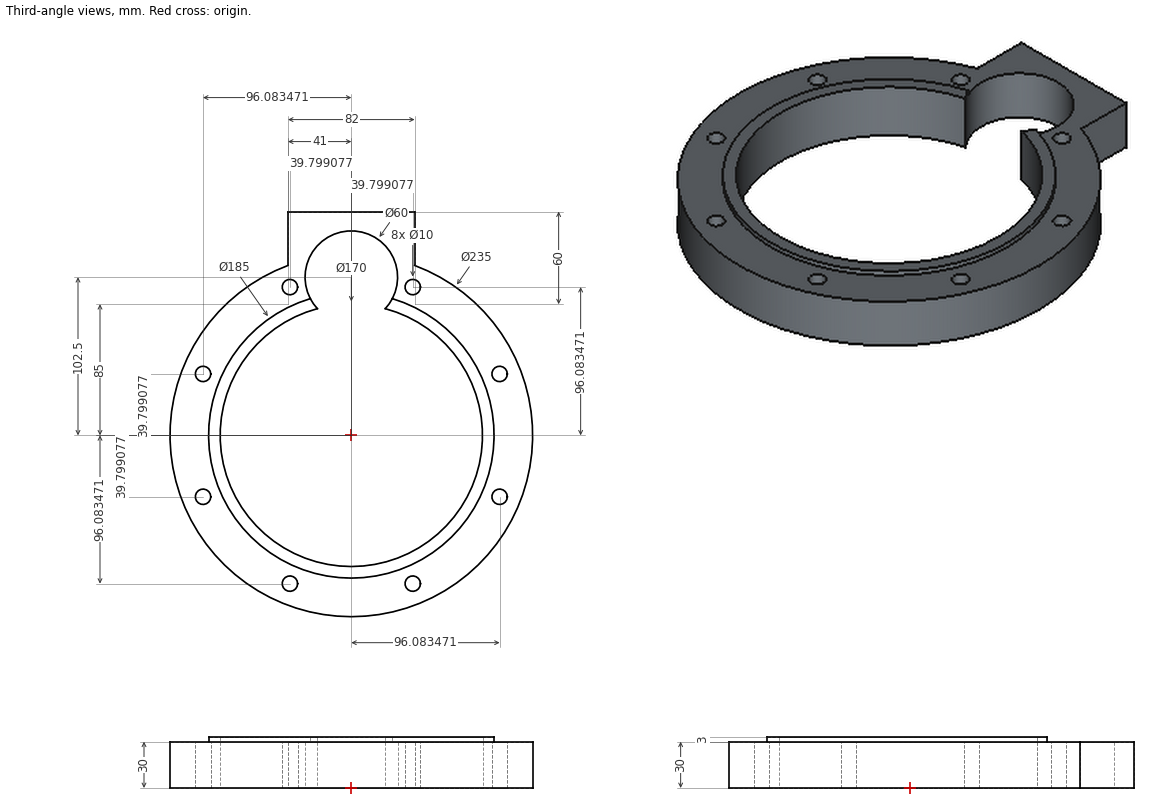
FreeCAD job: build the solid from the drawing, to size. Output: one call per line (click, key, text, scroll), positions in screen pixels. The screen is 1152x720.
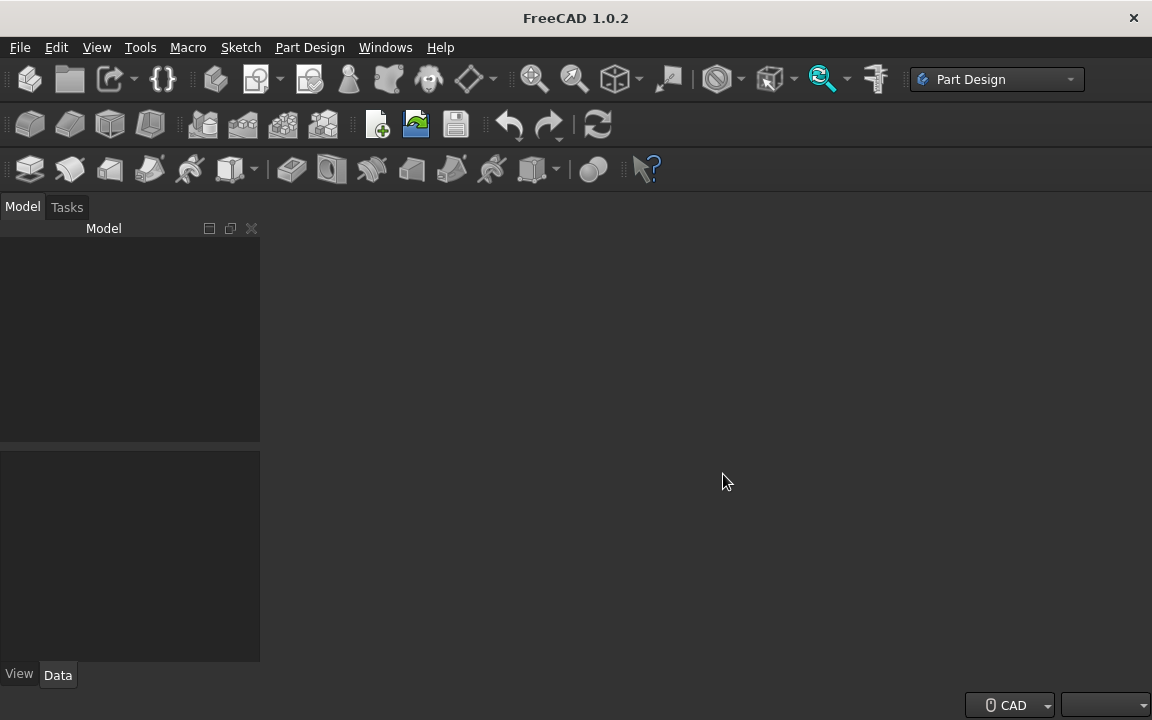
click(376, 124)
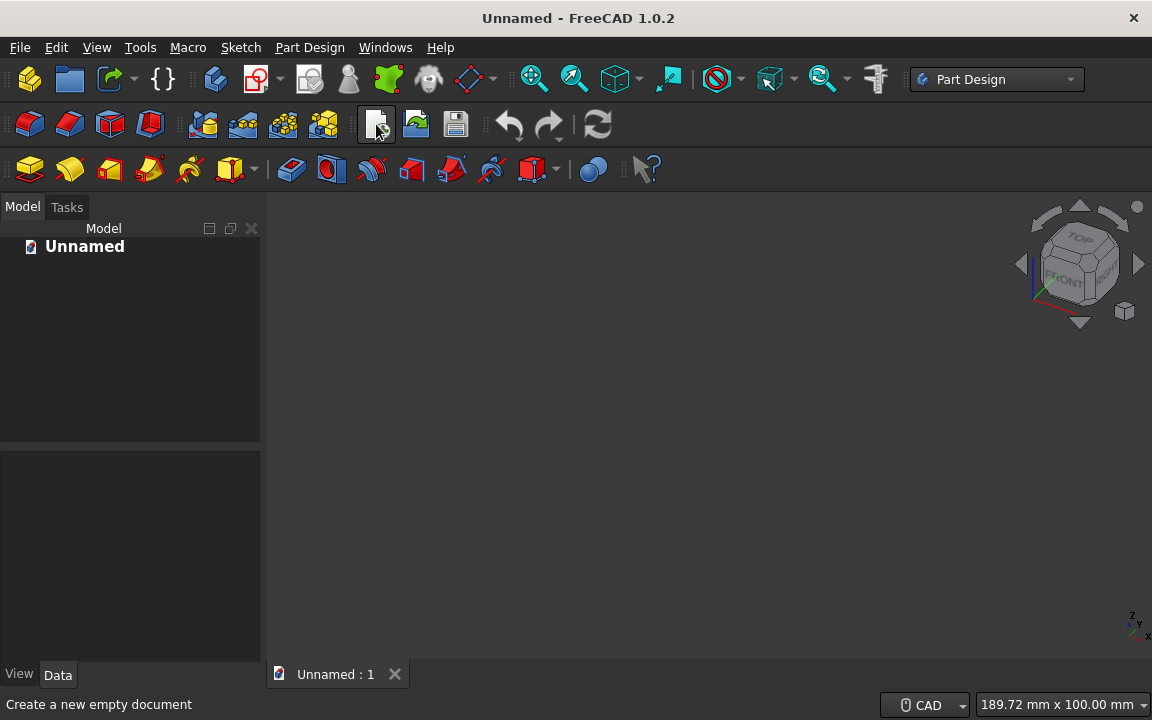
click(256, 80)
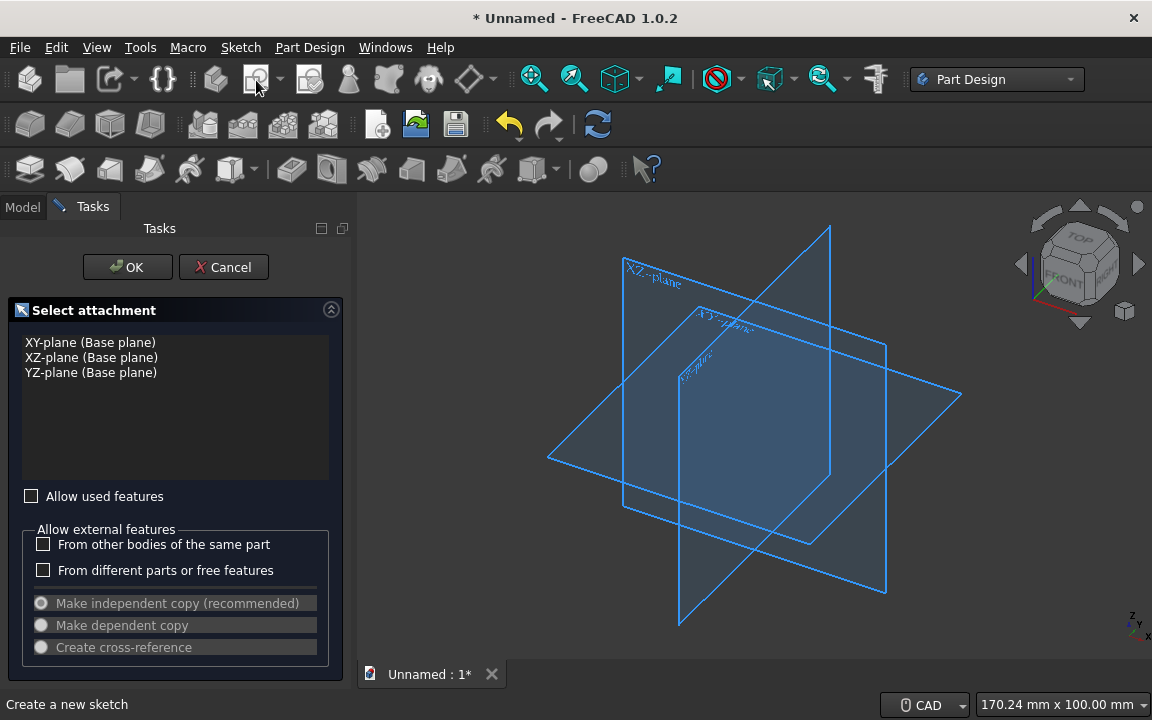
click(82, 342)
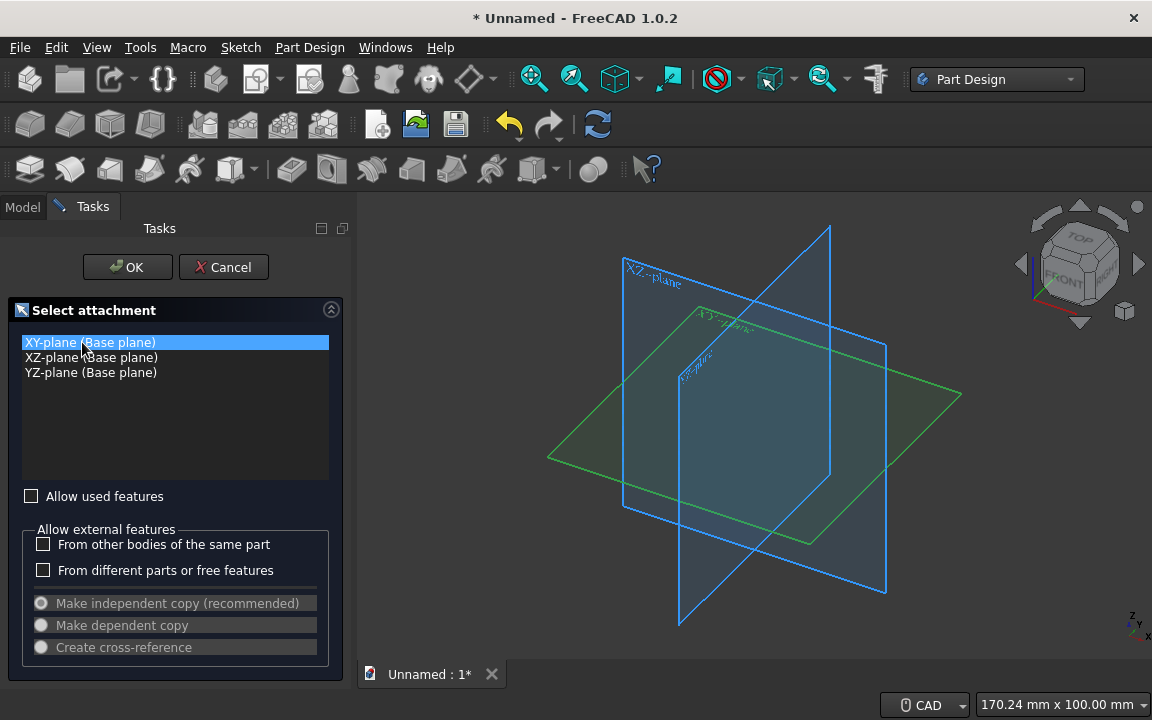
click(128, 267)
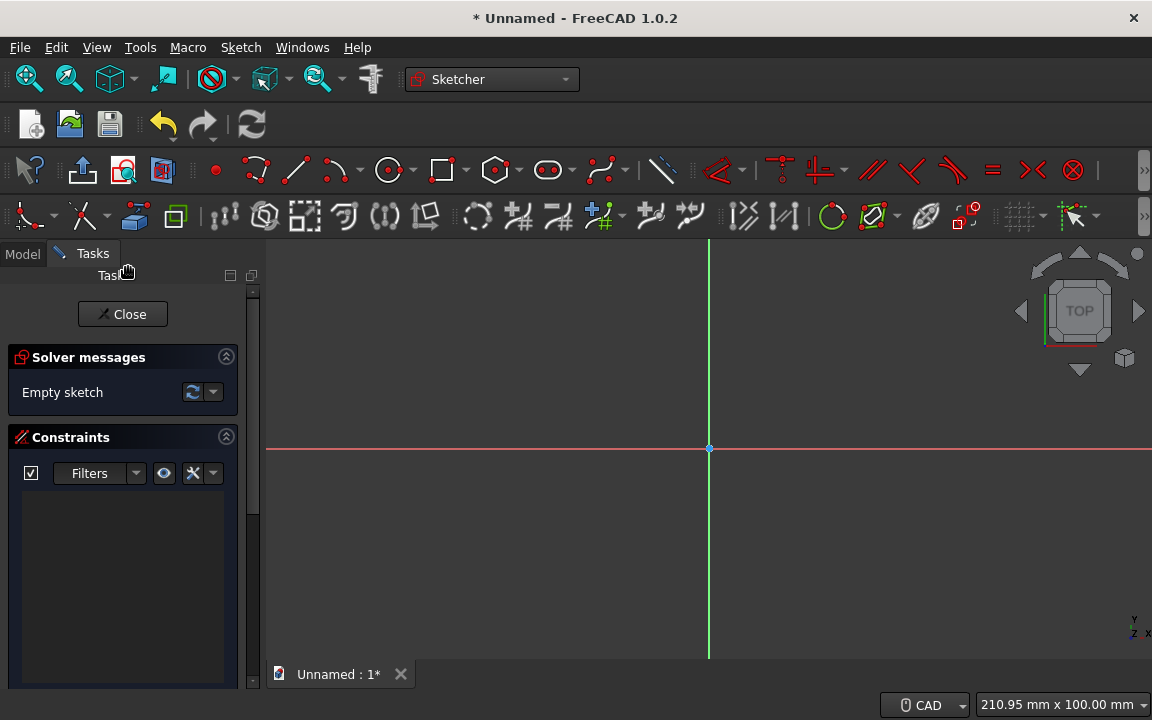
scroll(618, 449, down, 7)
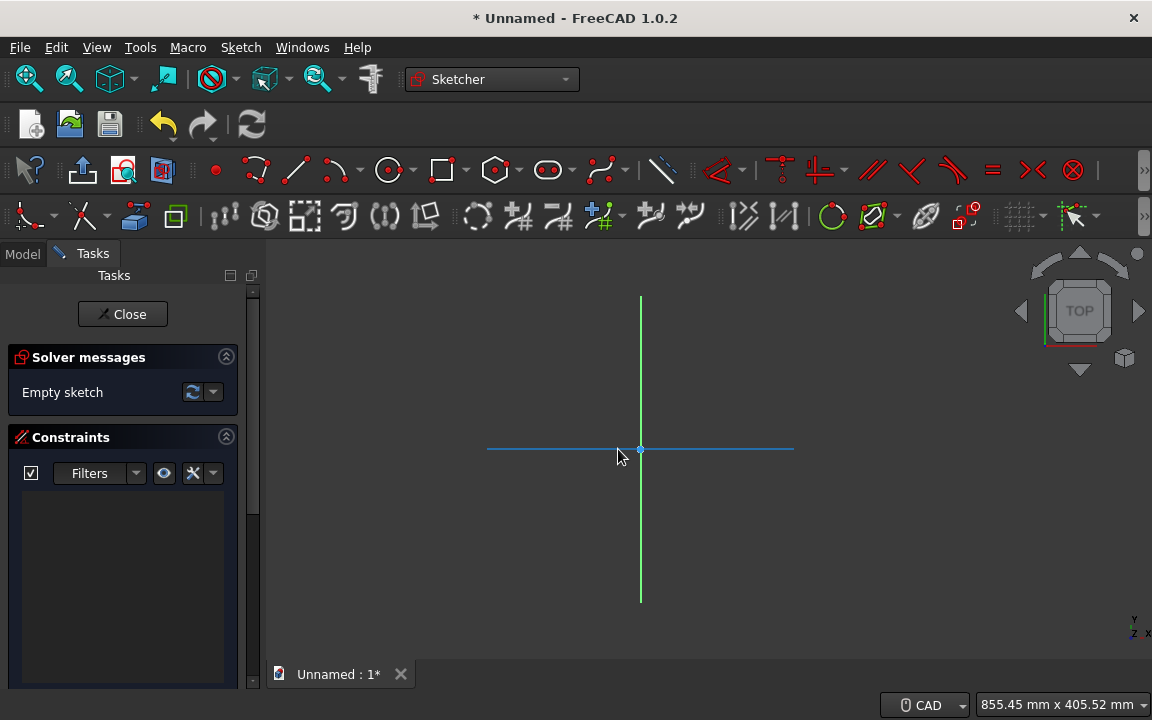
key(g)
key(c)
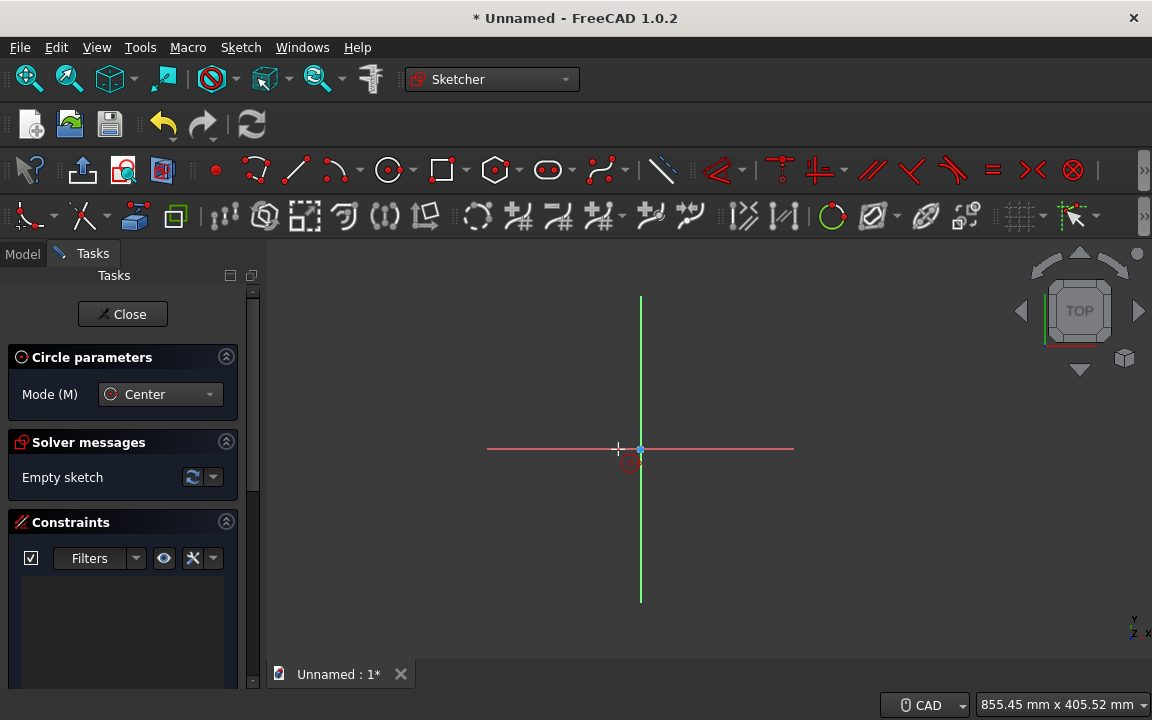
click(641, 449)
move(727, 363)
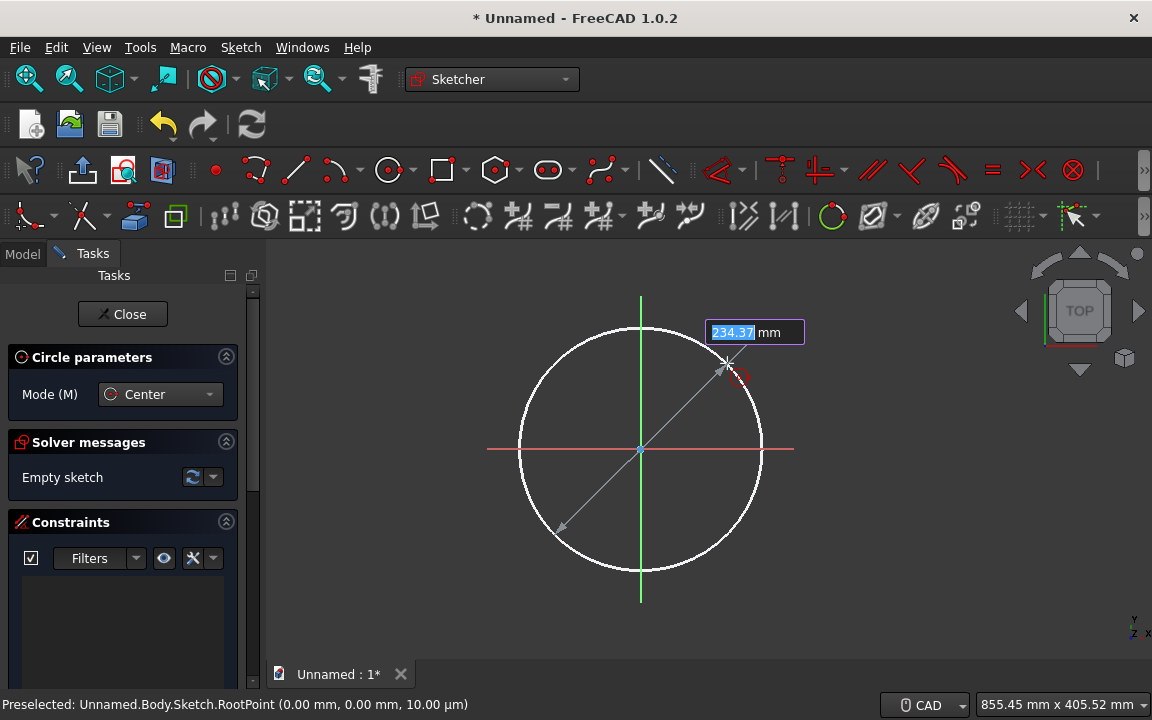
text(235)
key(Return)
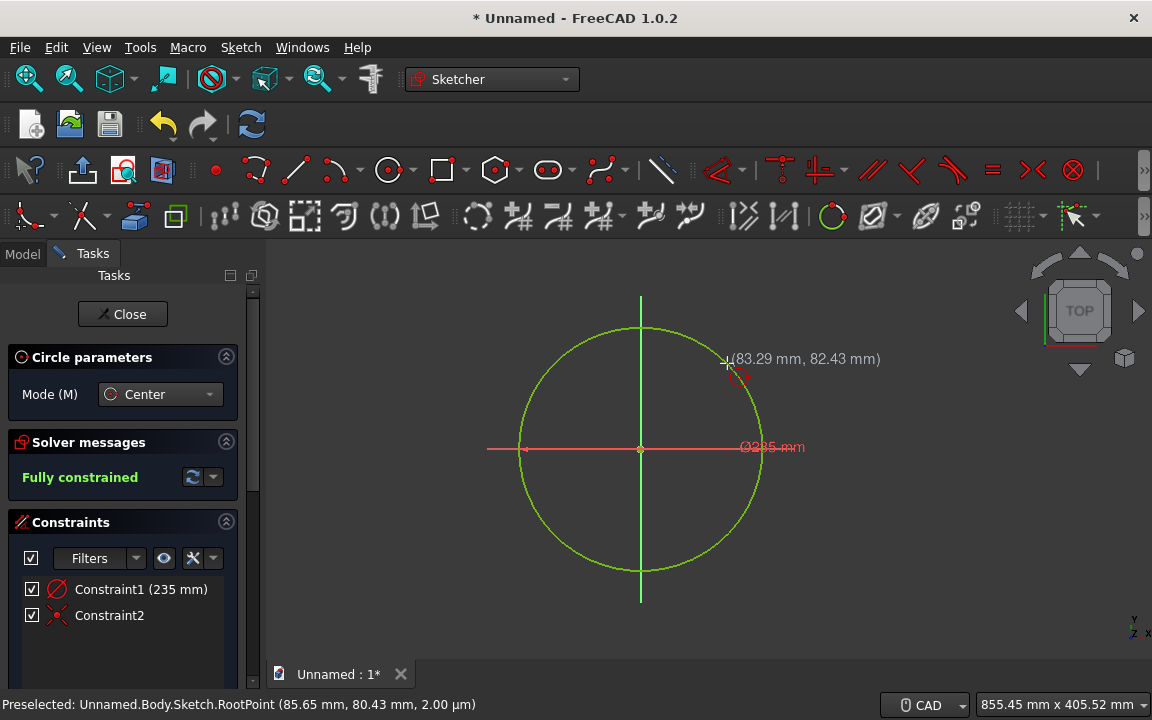
click(641, 449)
move(703, 387)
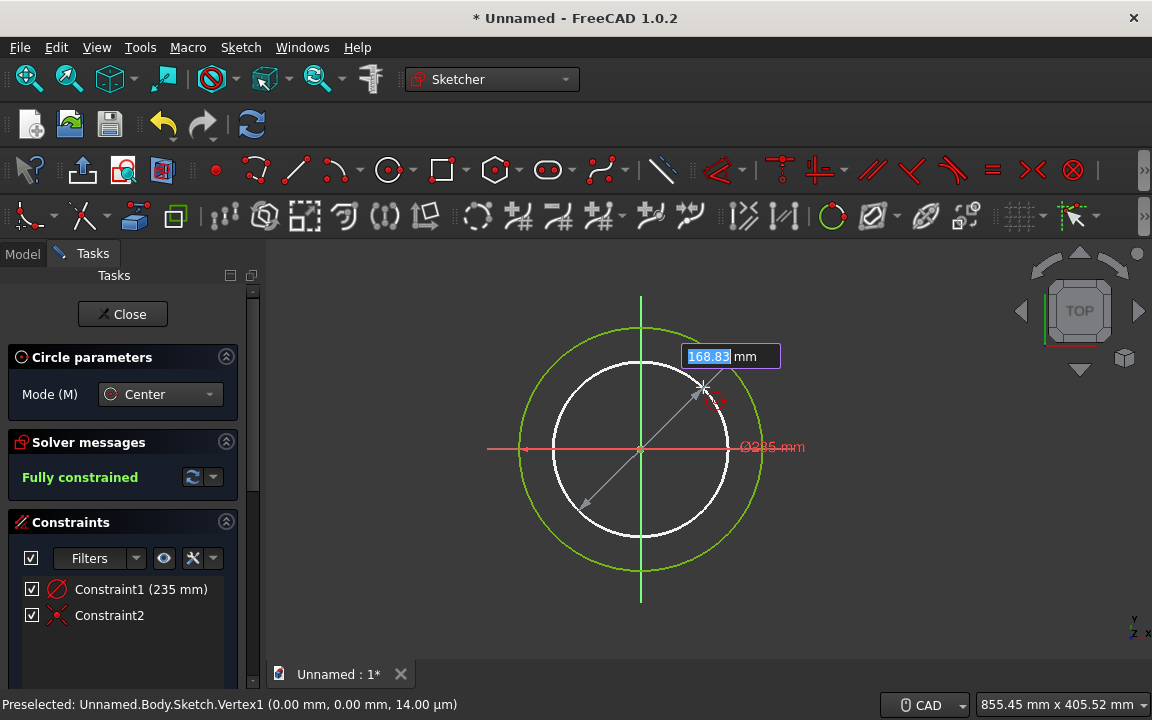
text(170)
key(Return)
key(Escape)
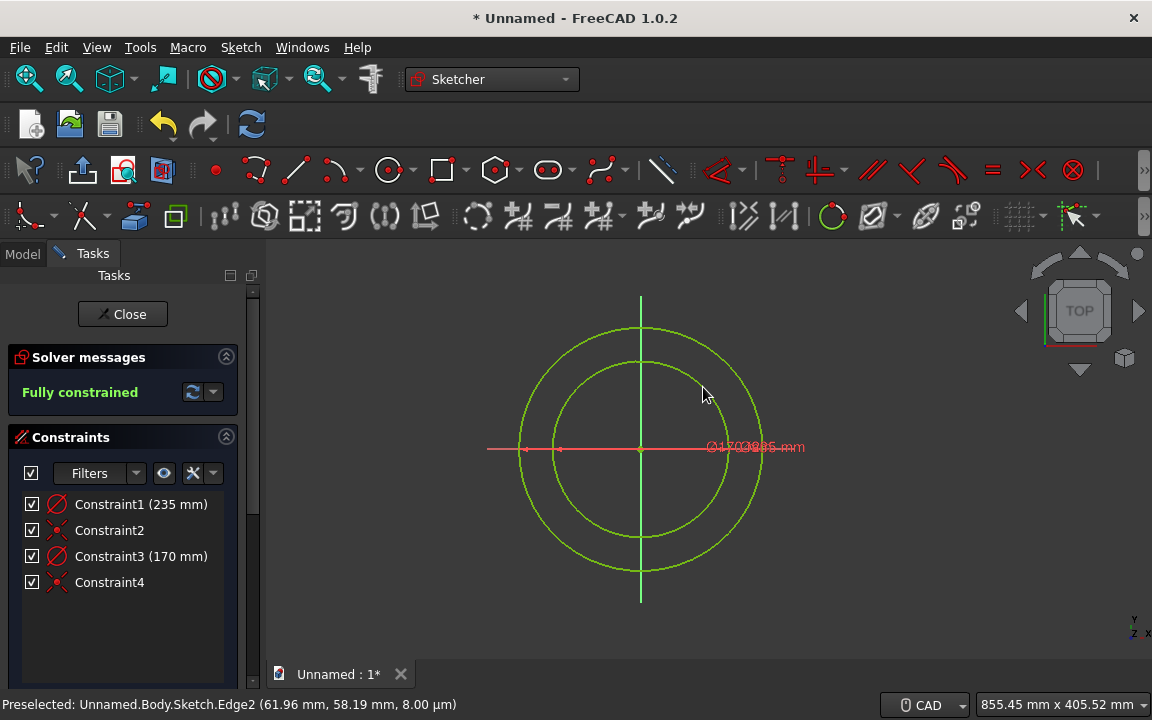
click(123, 314)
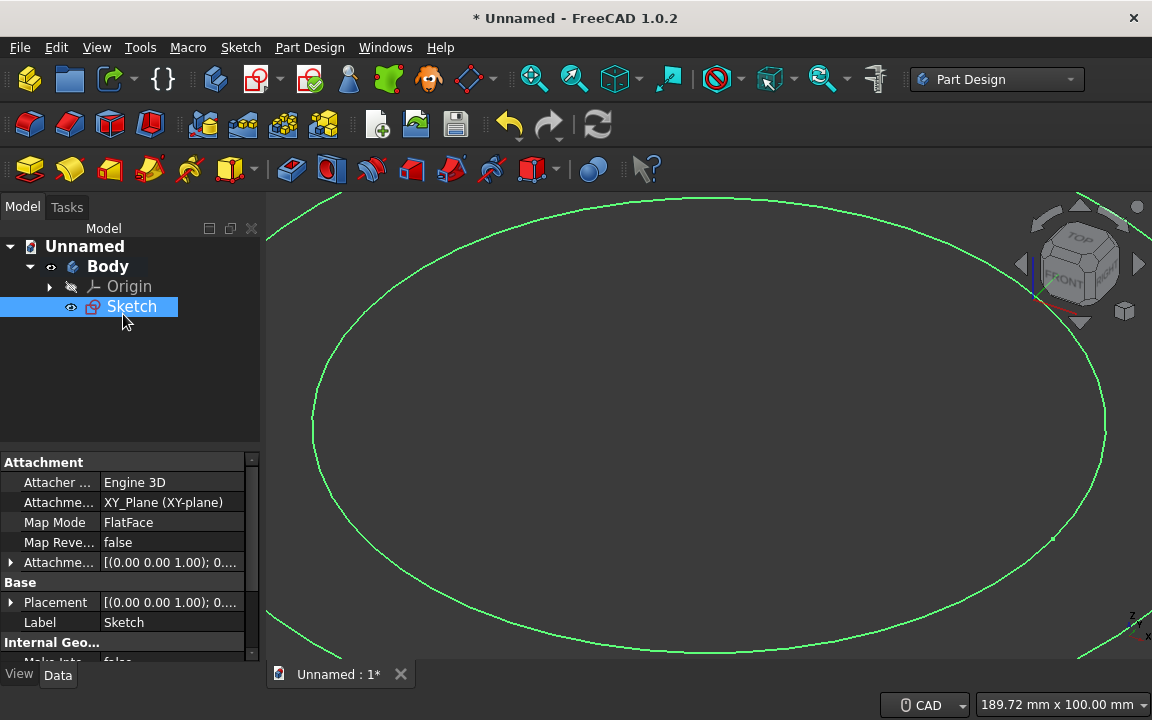
click(30, 170)